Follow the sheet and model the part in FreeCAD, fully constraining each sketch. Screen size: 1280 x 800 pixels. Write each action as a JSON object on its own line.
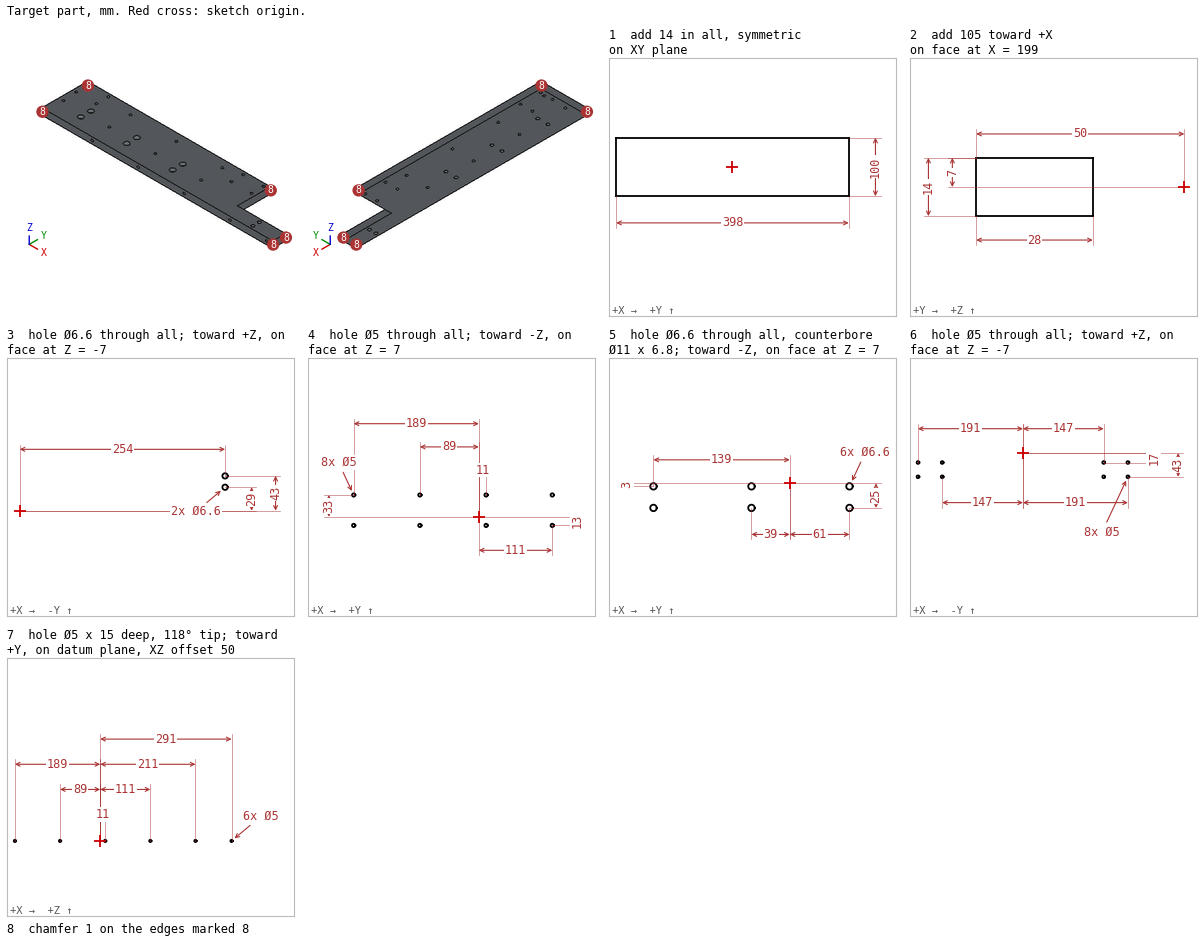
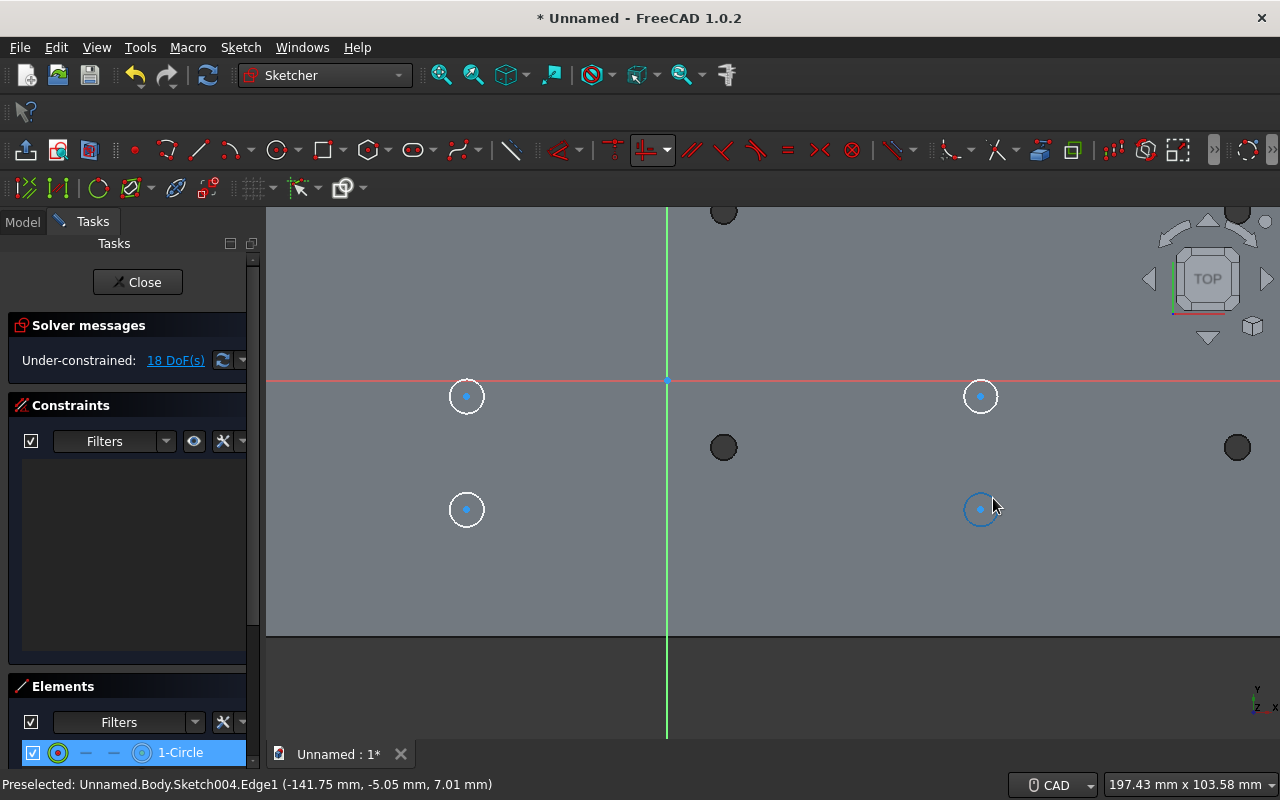
{"action": "left_click", "coordinate": [993, 498]}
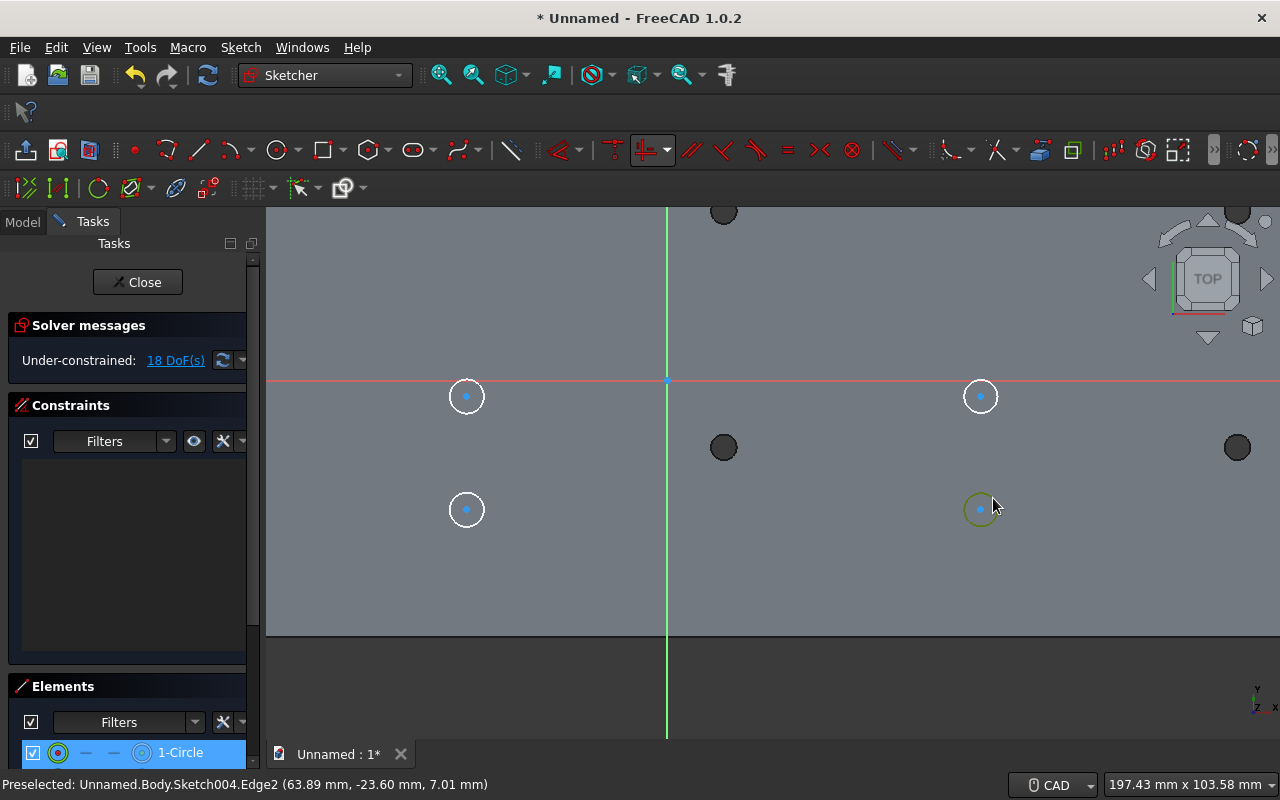
{"action": "left_click", "coordinate": [969, 408]}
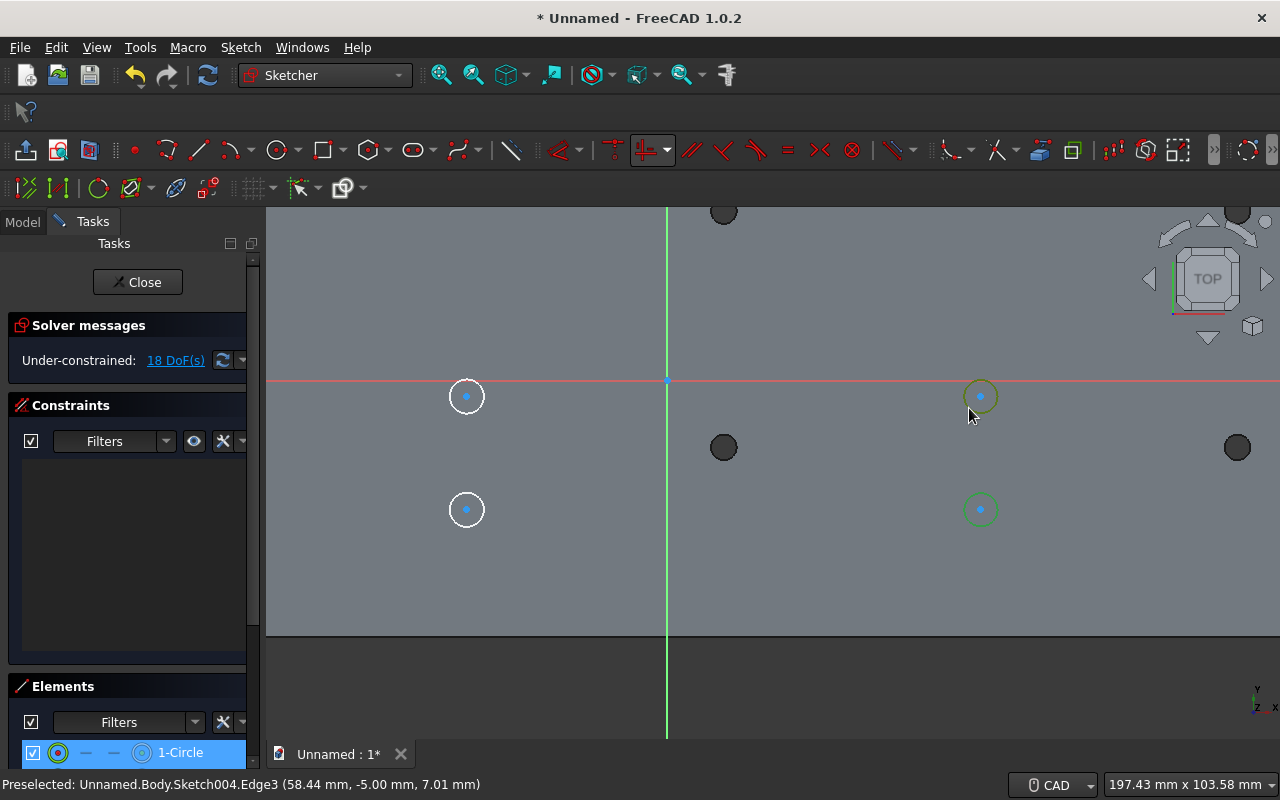
{"action": "left_click", "coordinate": [479, 498]}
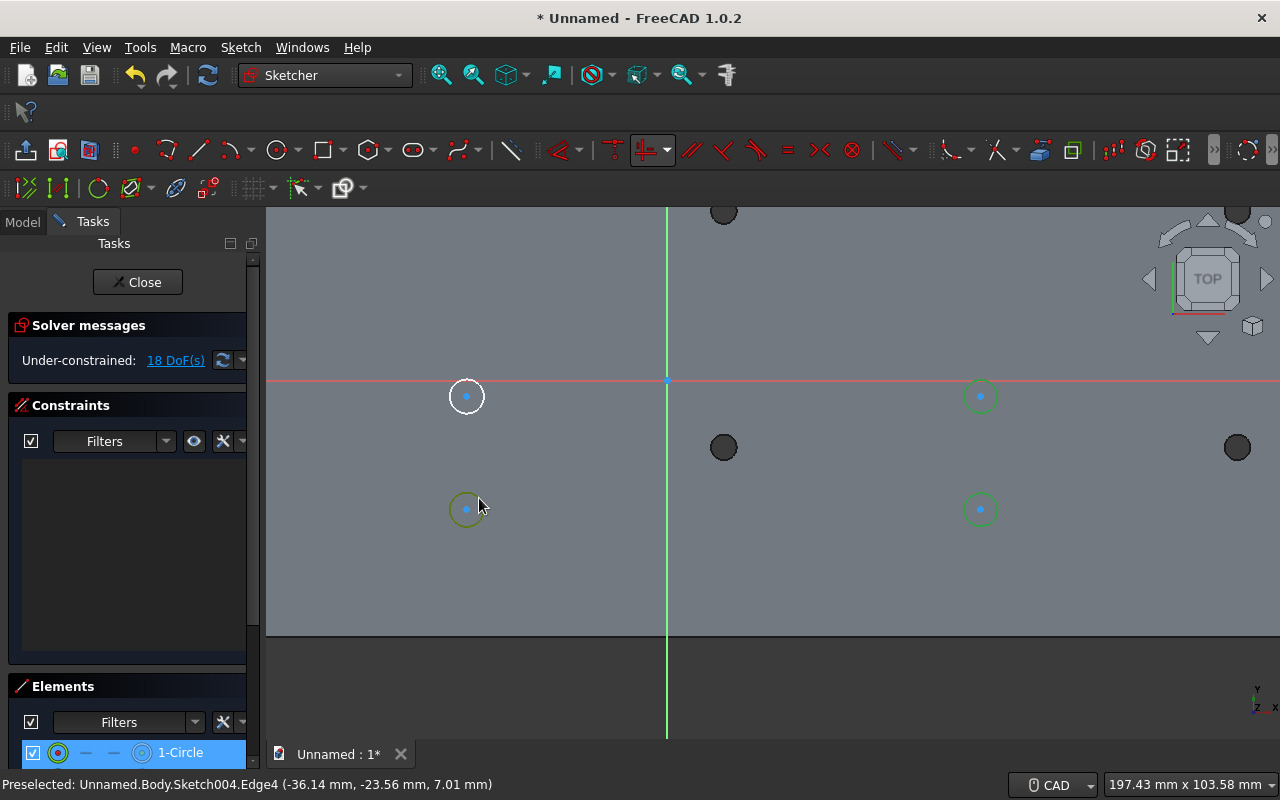
{"action": "left_click", "coordinate": [479, 384]}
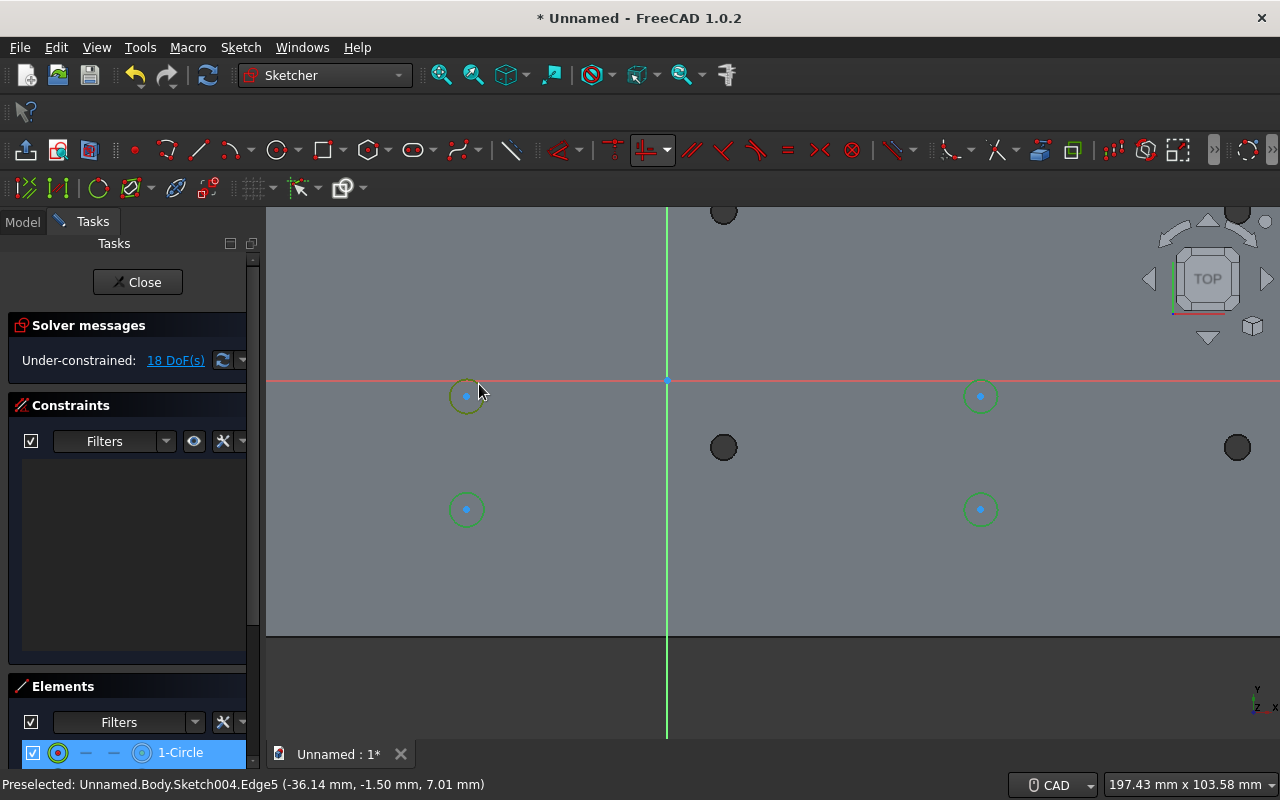
{"action": "scroll", "coordinate": [993, 498], "scroll_direction": "down", "scroll_amount": 3}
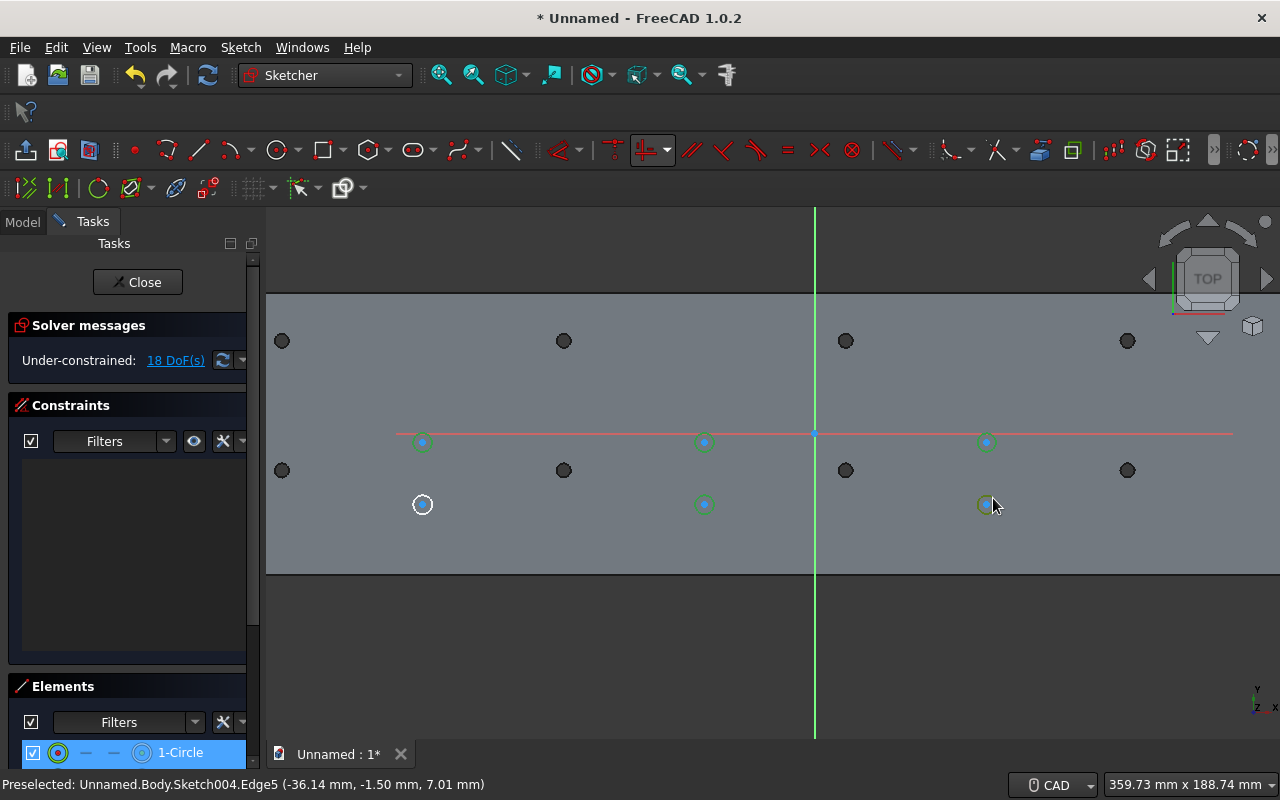
{"action": "scroll", "coordinate": [429, 498], "scroll_direction": "up", "scroll_amount": 2}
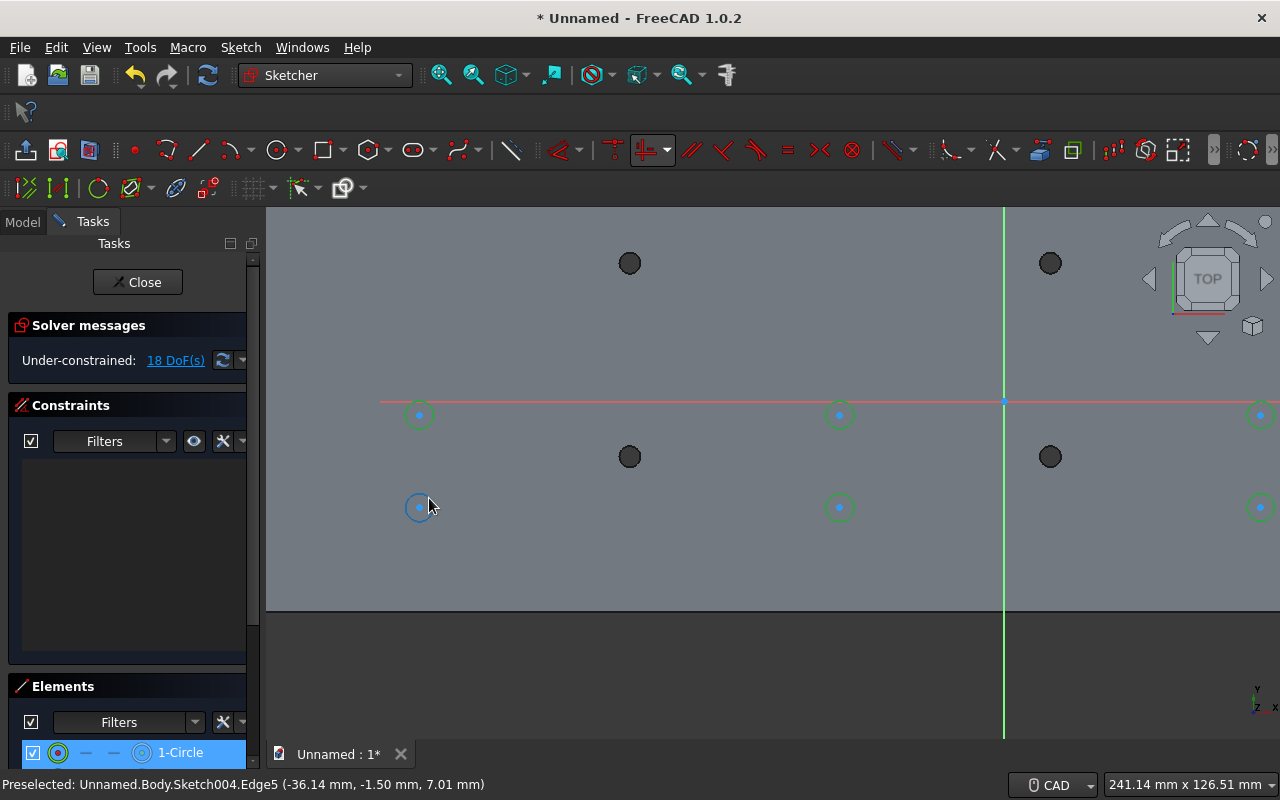
{"action": "left_click", "coordinate": [429, 498]}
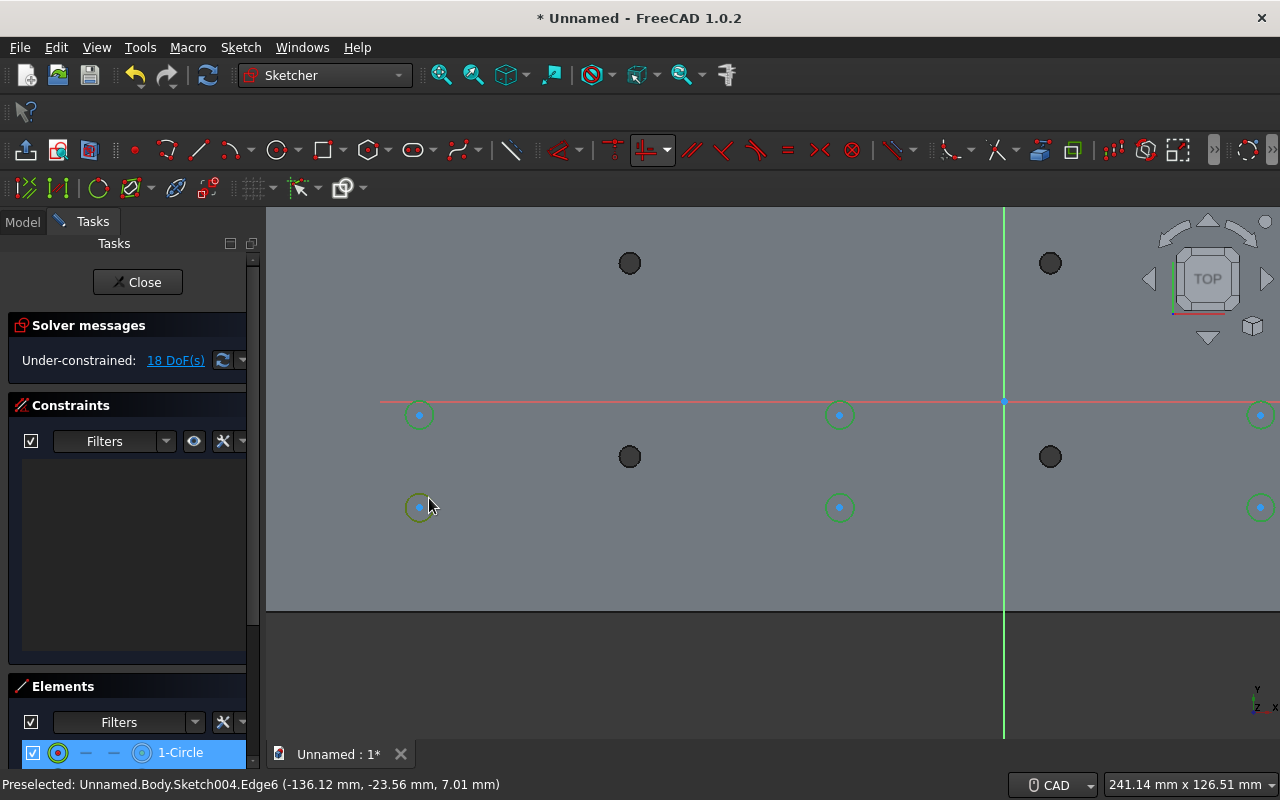
{"action": "left_click", "coordinate": [788, 150]}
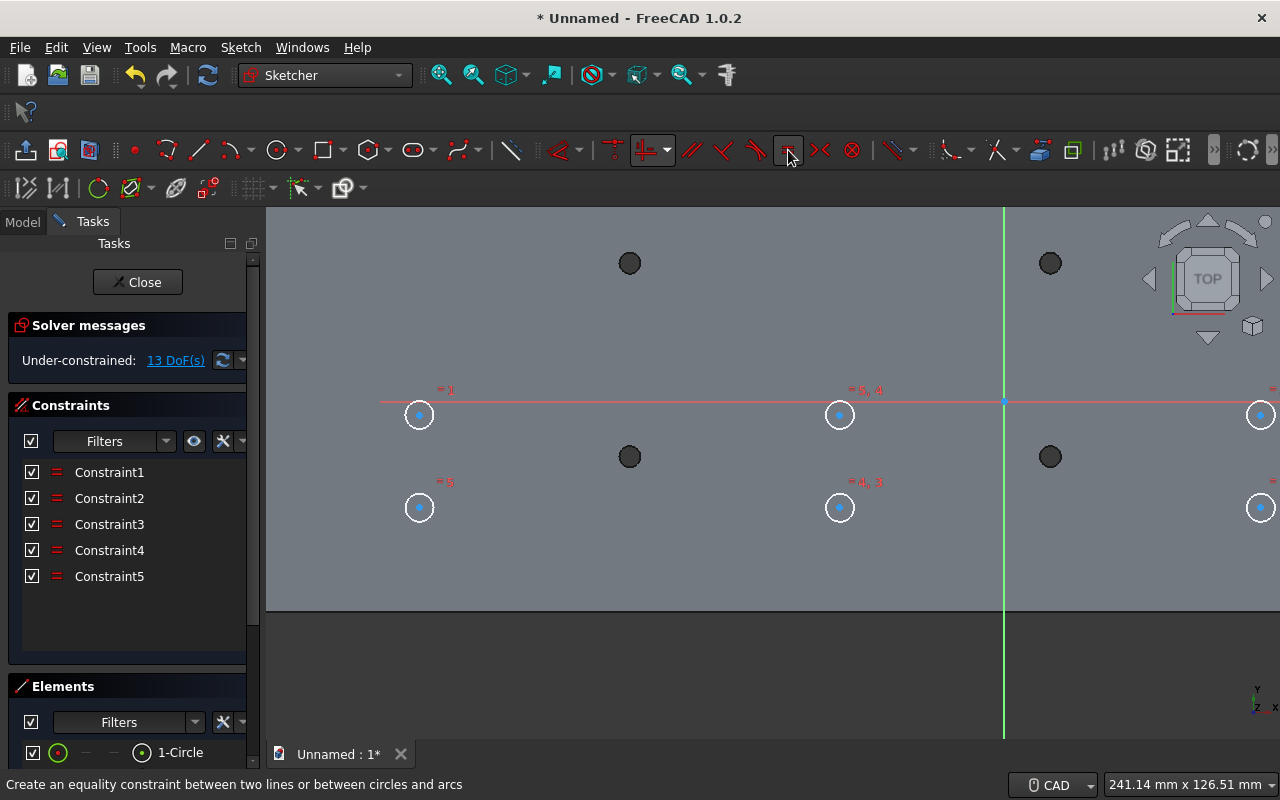
{"action": "scroll", "coordinate": [429, 498], "scroll_direction": "down", "scroll_amount": 2}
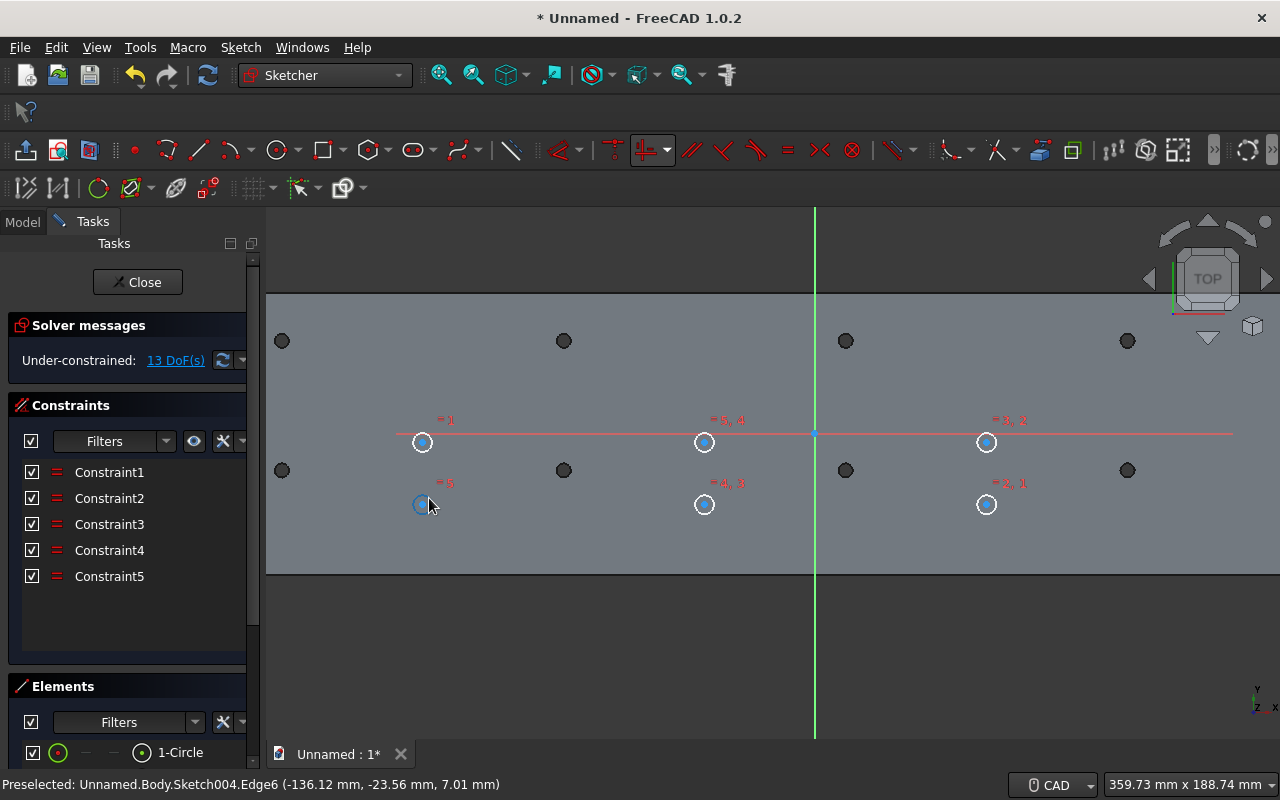
{"action": "left_click", "coordinate": [987, 505]}